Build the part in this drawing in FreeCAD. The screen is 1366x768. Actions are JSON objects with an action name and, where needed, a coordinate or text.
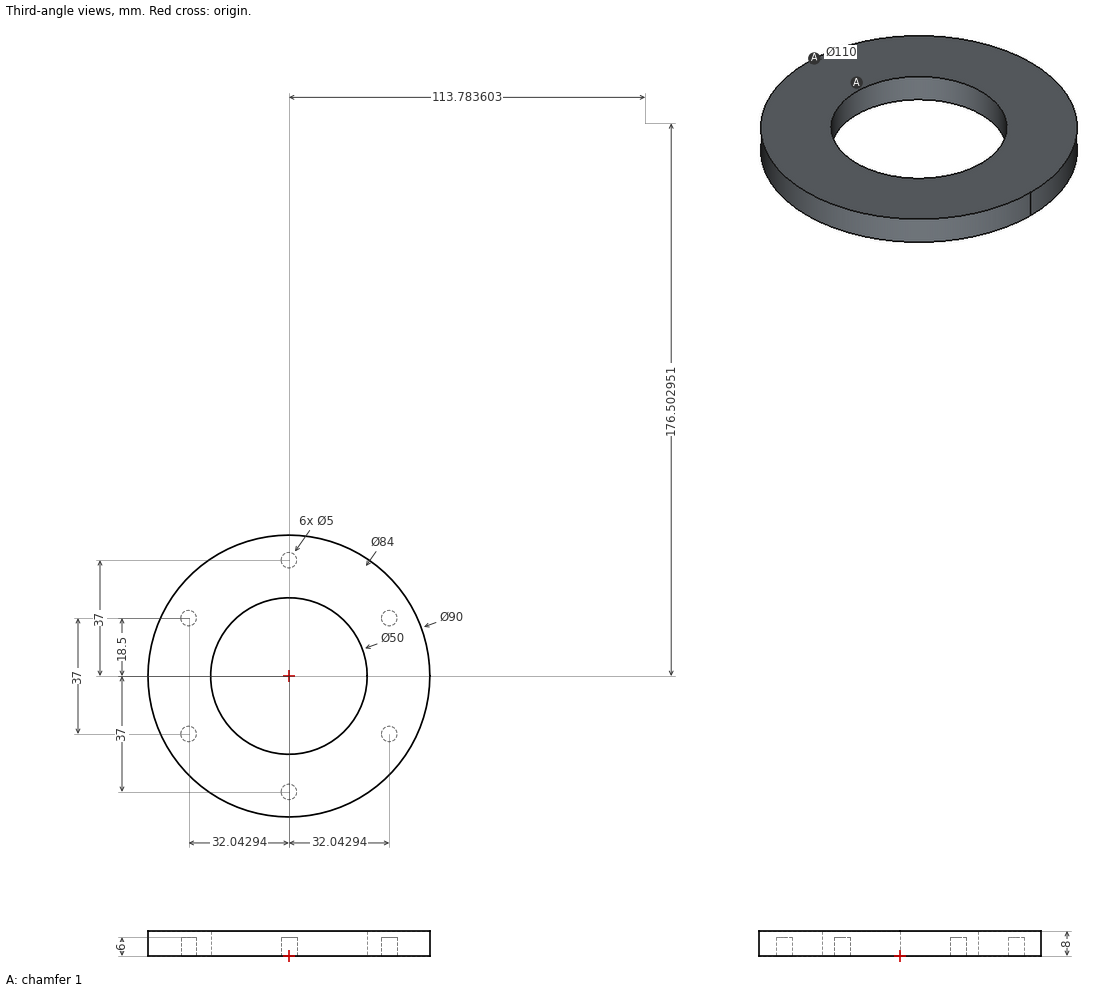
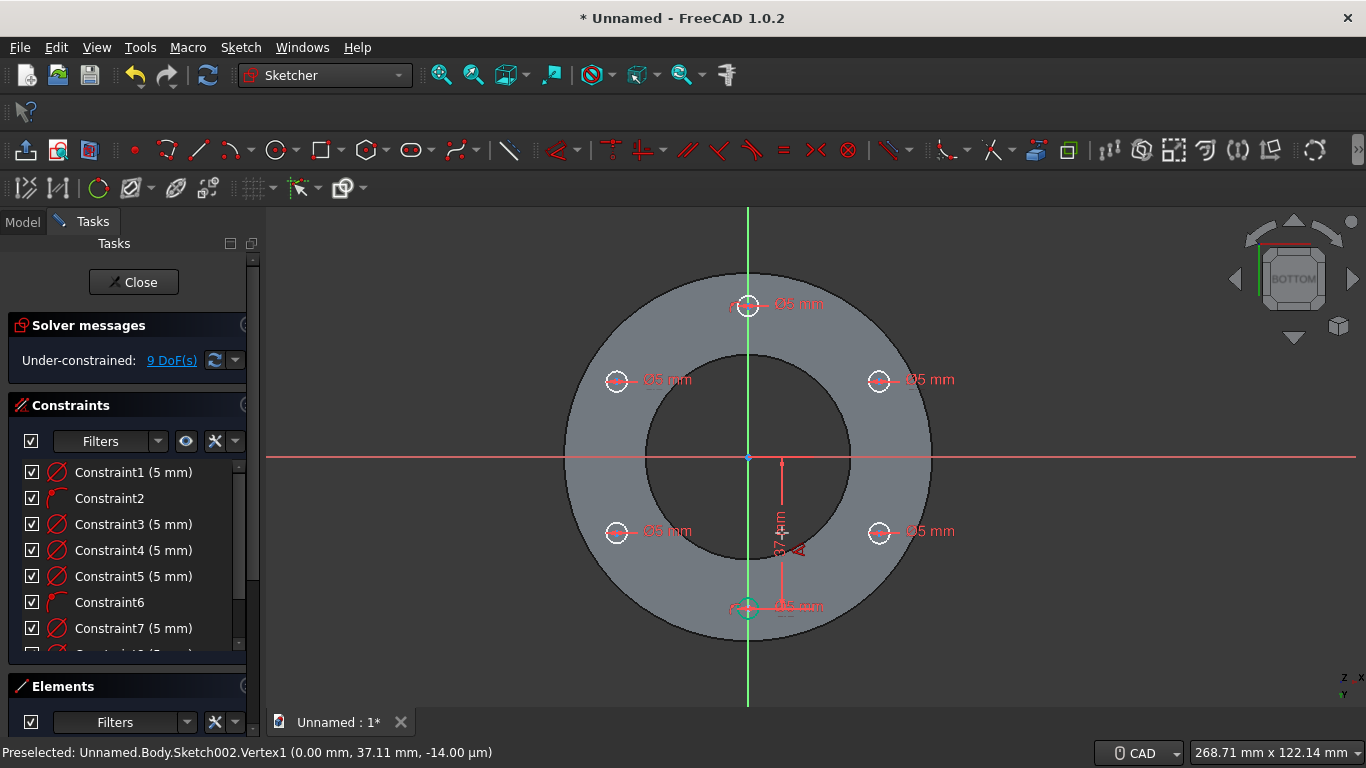
{"action": "left_click", "coordinate": [748, 306]}
{"action": "left_click", "coordinate": [782, 382]}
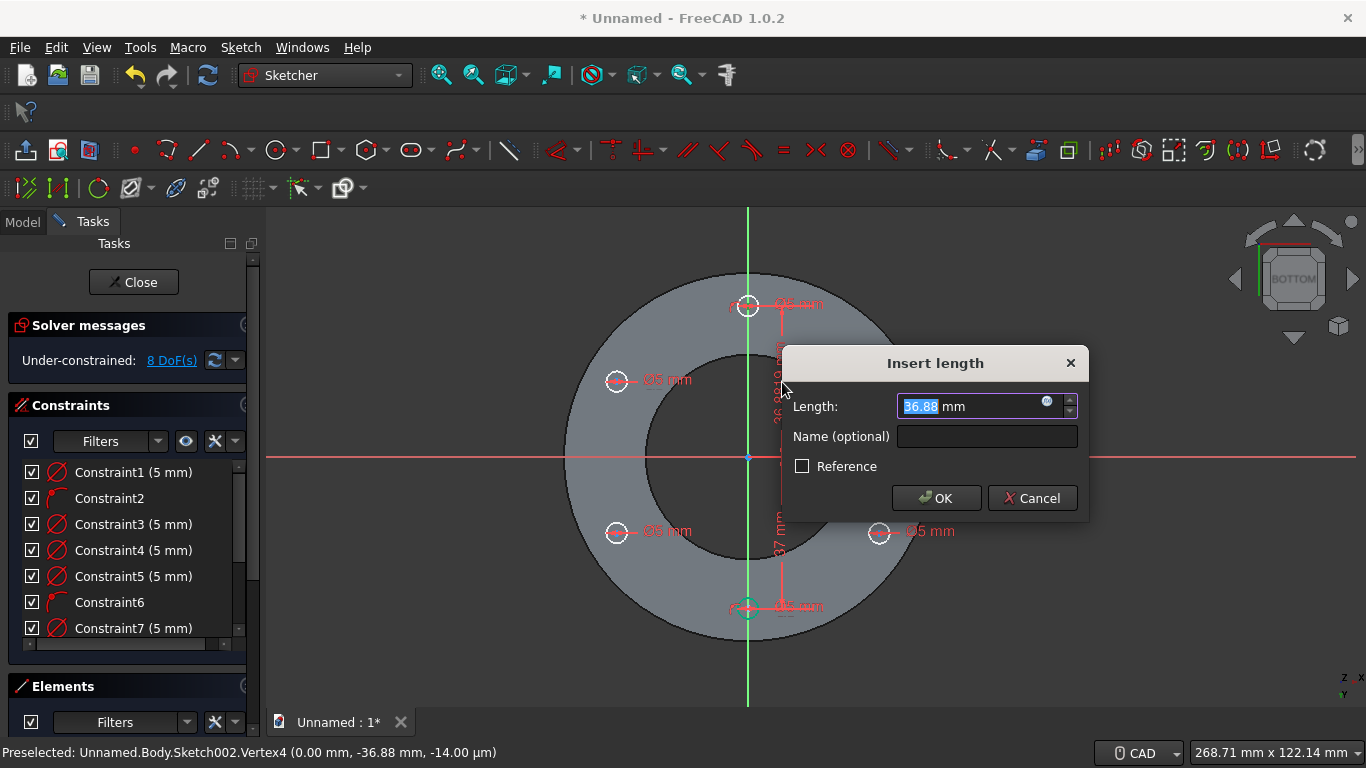
{"action": "type", "text": "37"}
{"action": "key", "text": "Return"}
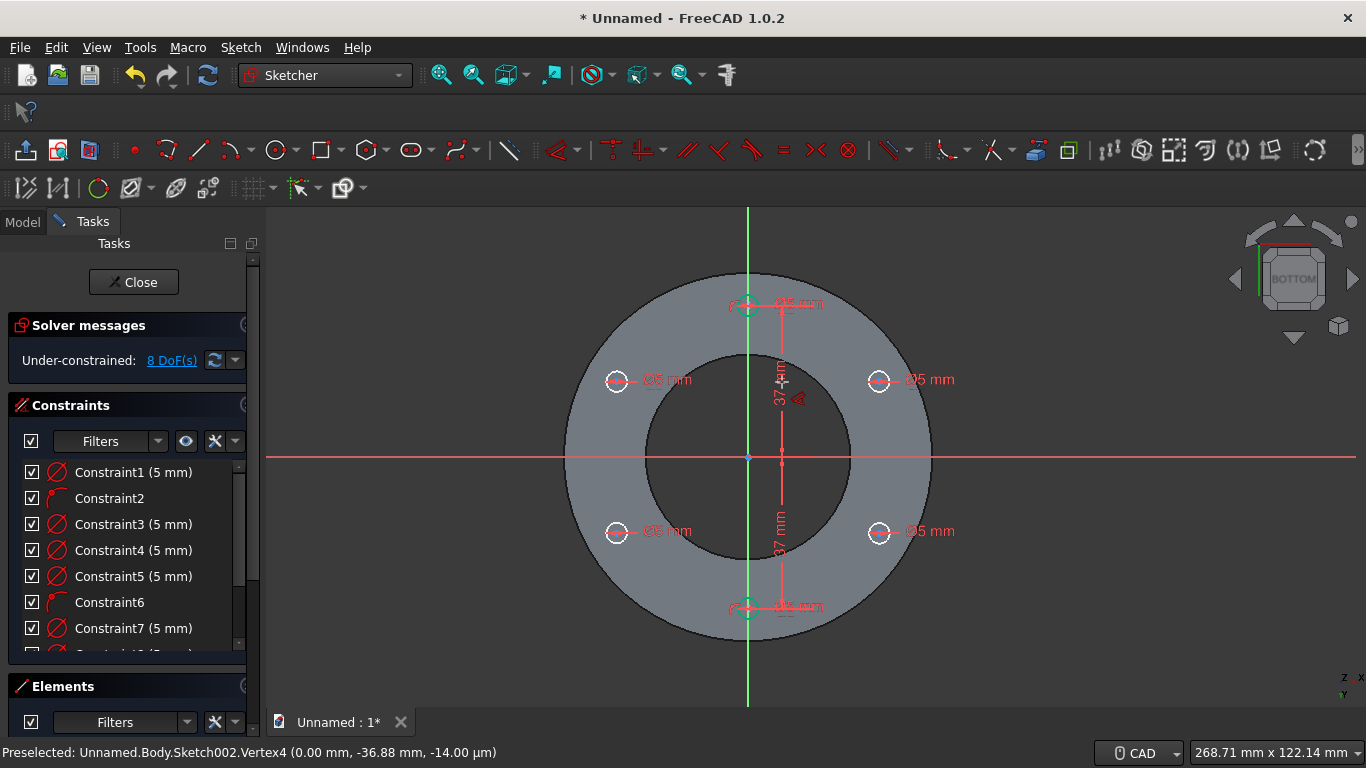
{"action": "left_click", "coordinate": [617, 533]}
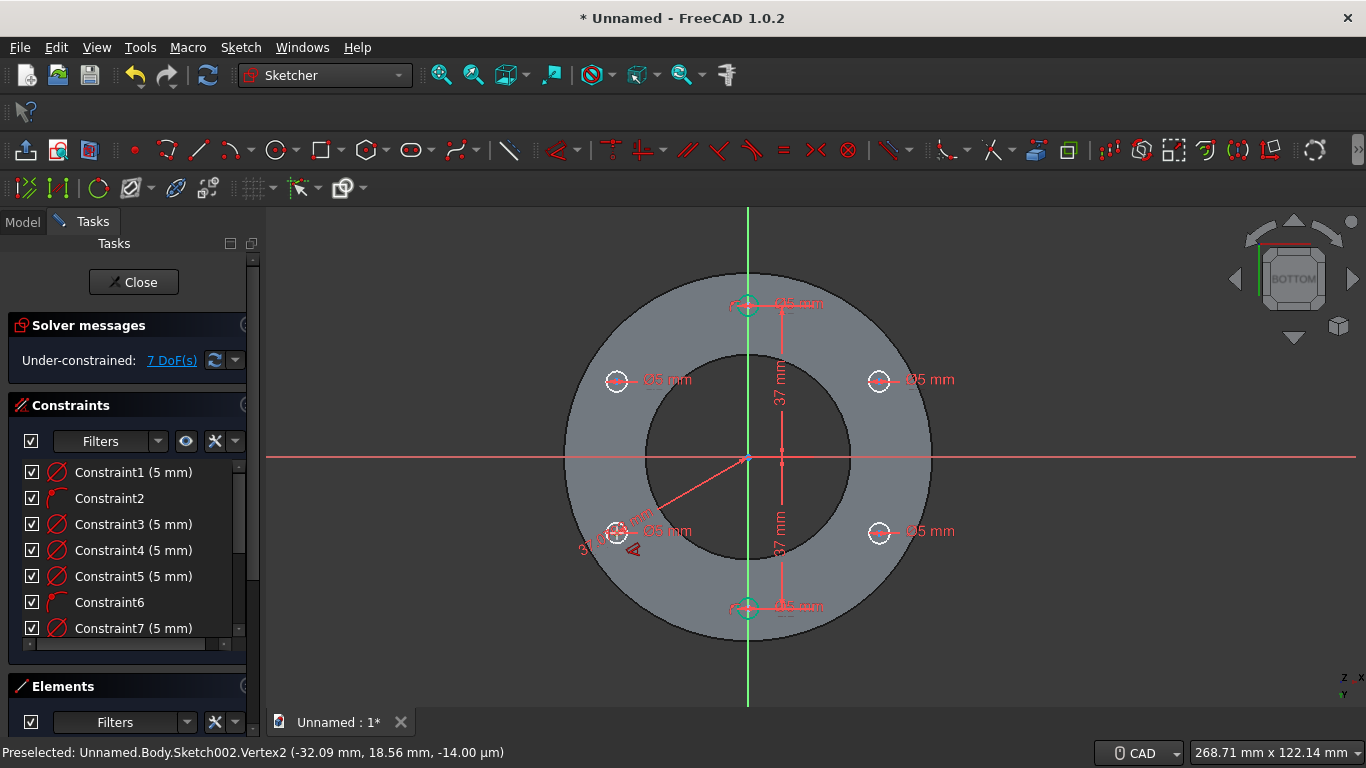
{"action": "left_click", "coordinate": [617, 382]}
{"action": "left_click", "coordinate": [583, 423]}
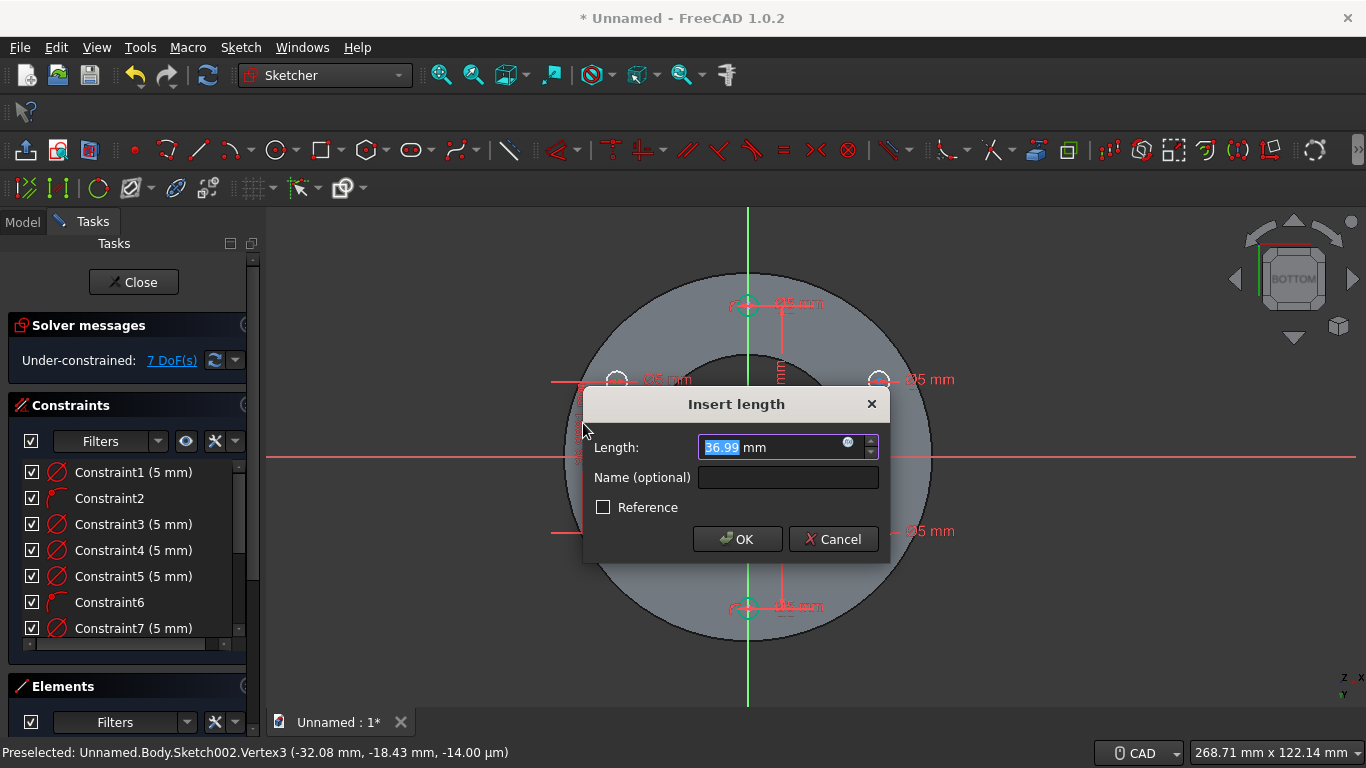
{"action": "type", "text": "37"}
{"action": "key", "text": "Return"}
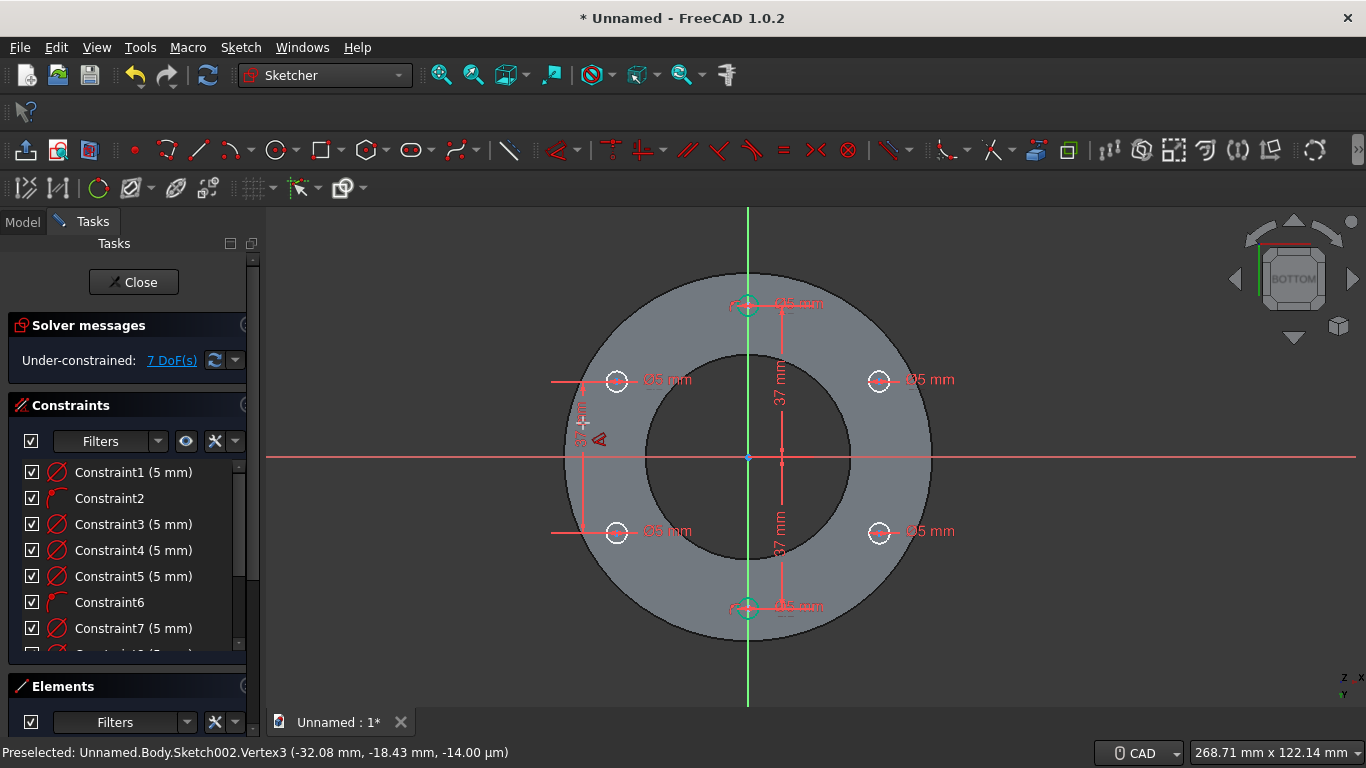
{"action": "left_click", "coordinate": [617, 533]}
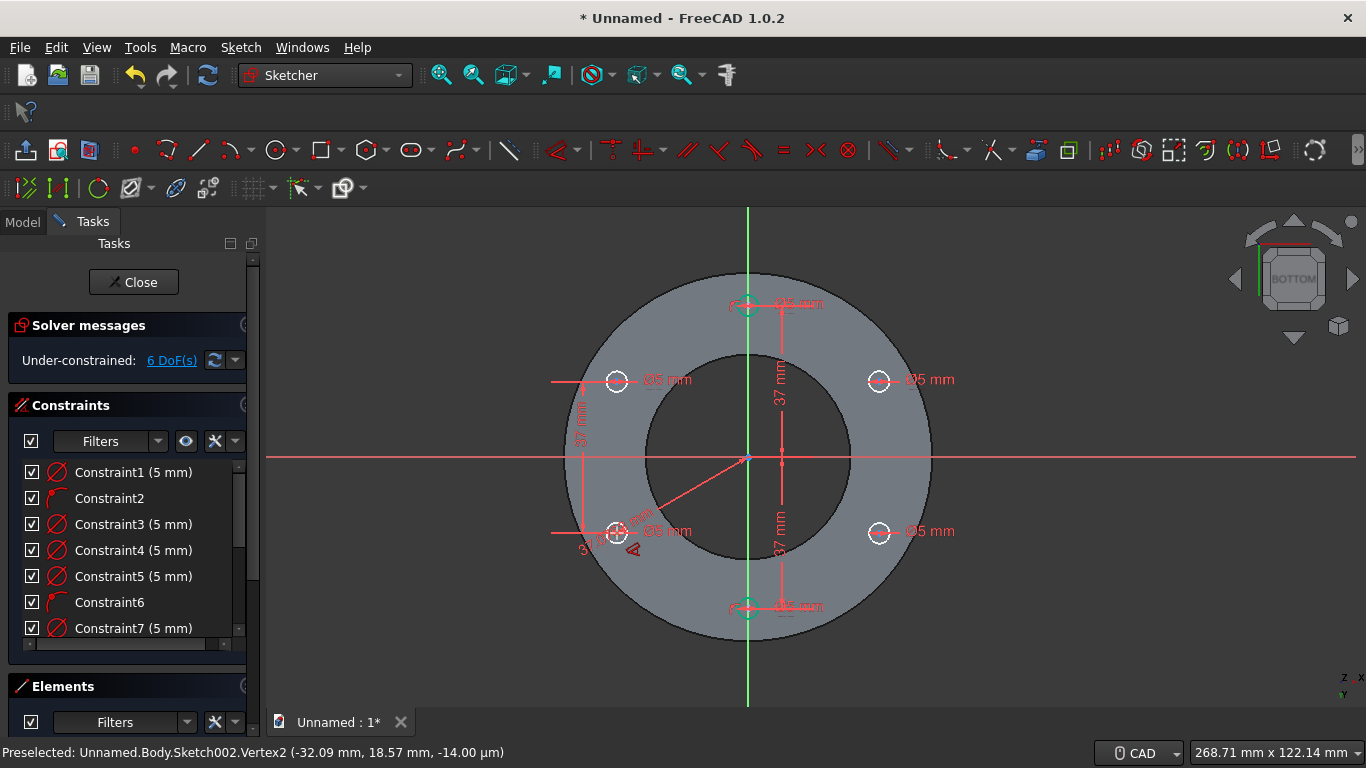
{"action": "left_click", "coordinate": [879, 382]}
{"action": "left_click", "coordinate": [583, 492]}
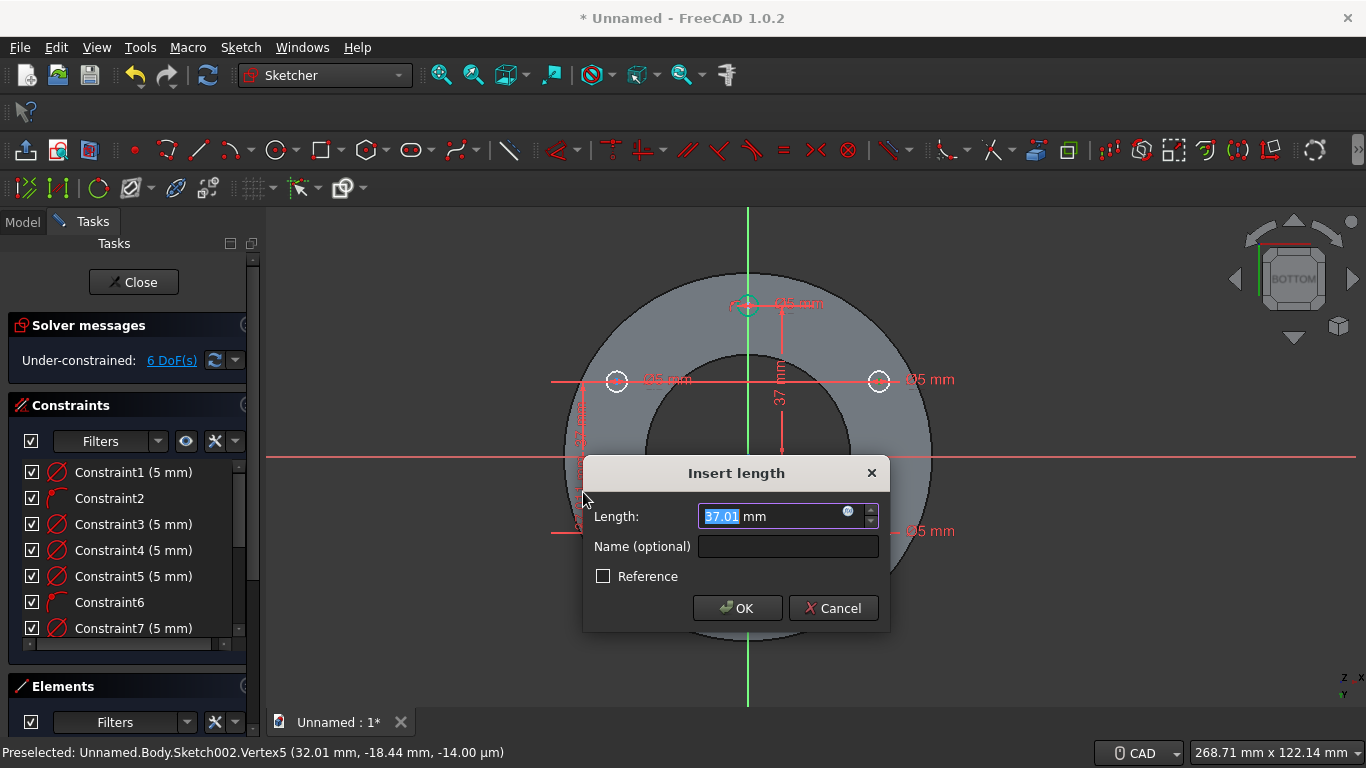
{"action": "type", "text": "37"}
{"action": "key", "text": "Return"}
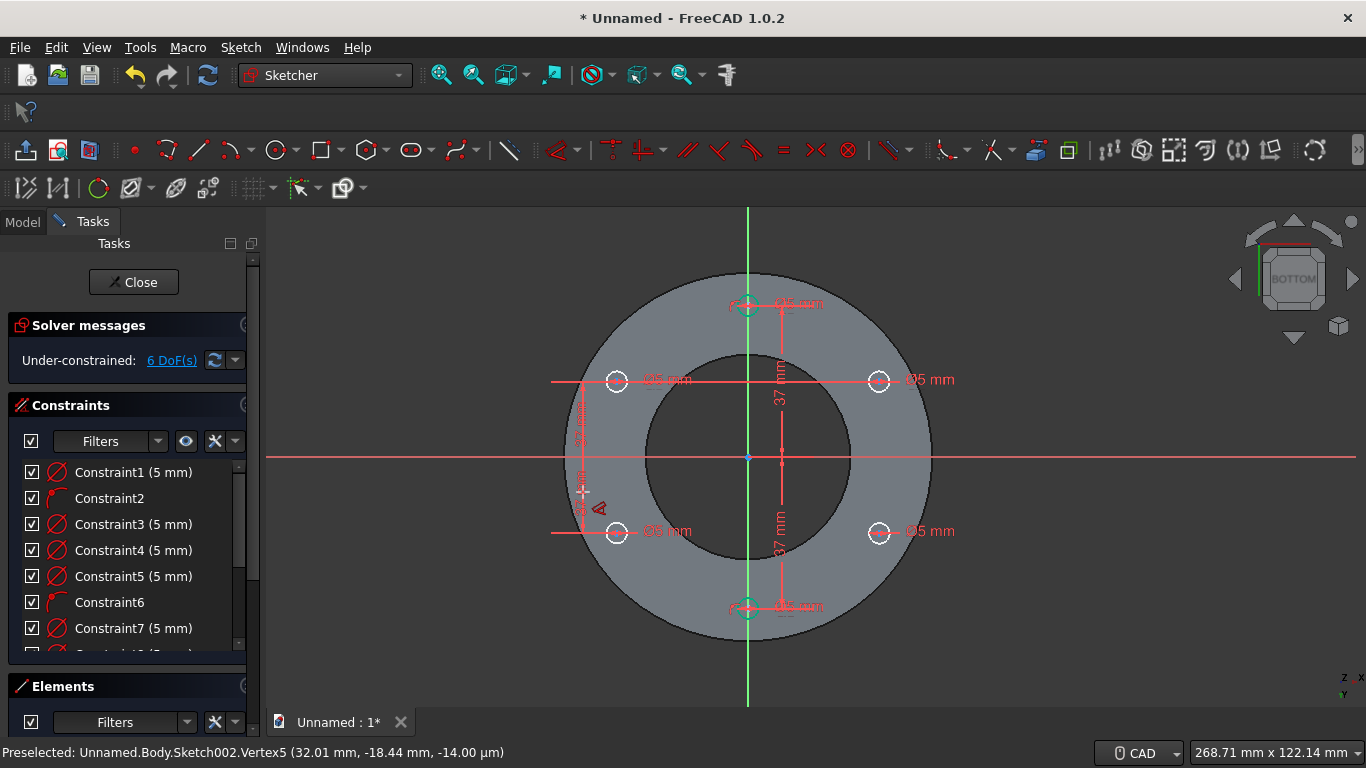
{"action": "left_click", "coordinate": [879, 382]}